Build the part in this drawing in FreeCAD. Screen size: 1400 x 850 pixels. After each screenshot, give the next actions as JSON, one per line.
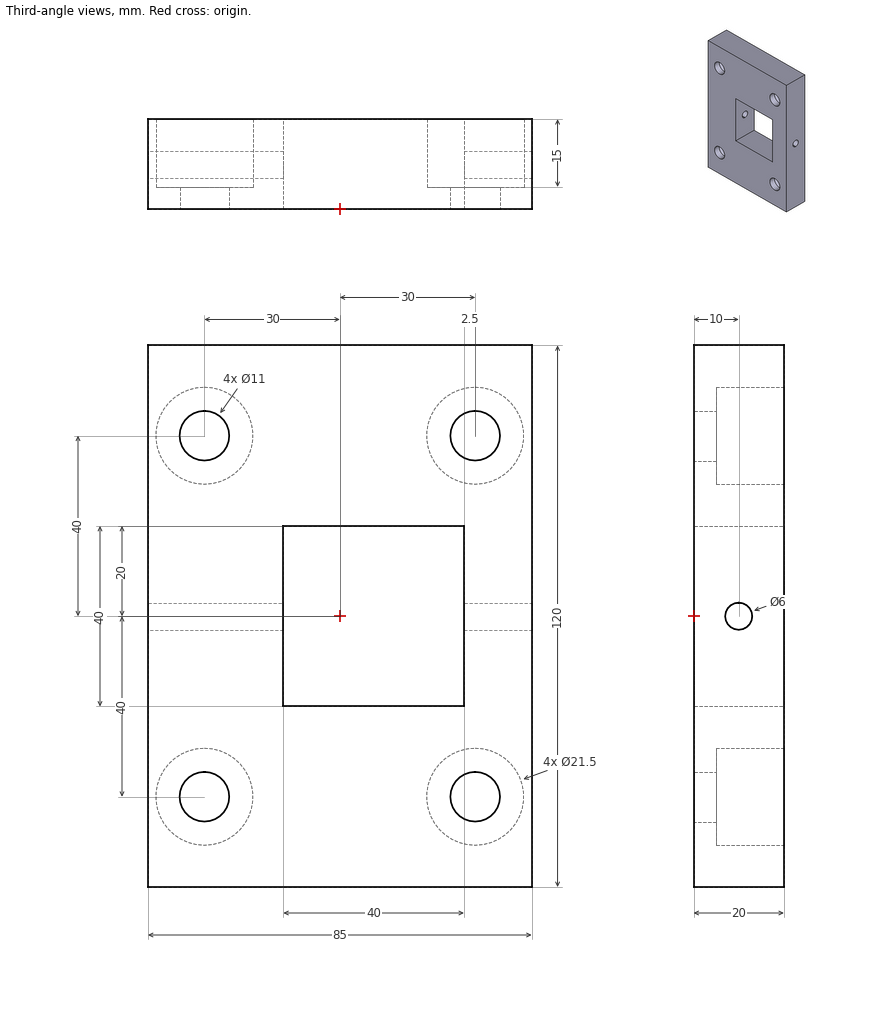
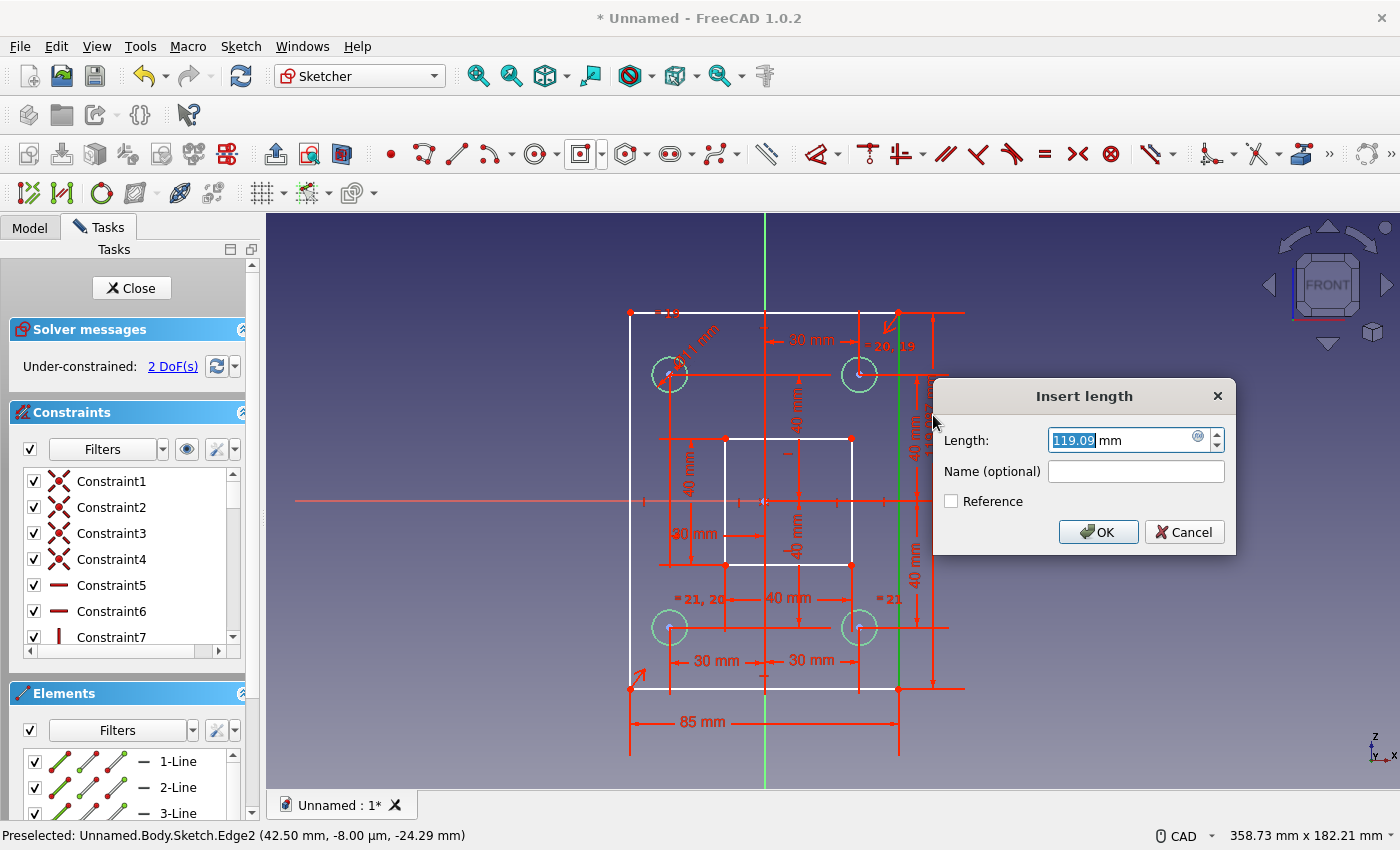
{"action": "type", "text": "120"}
{"action": "key", "text": "Return"}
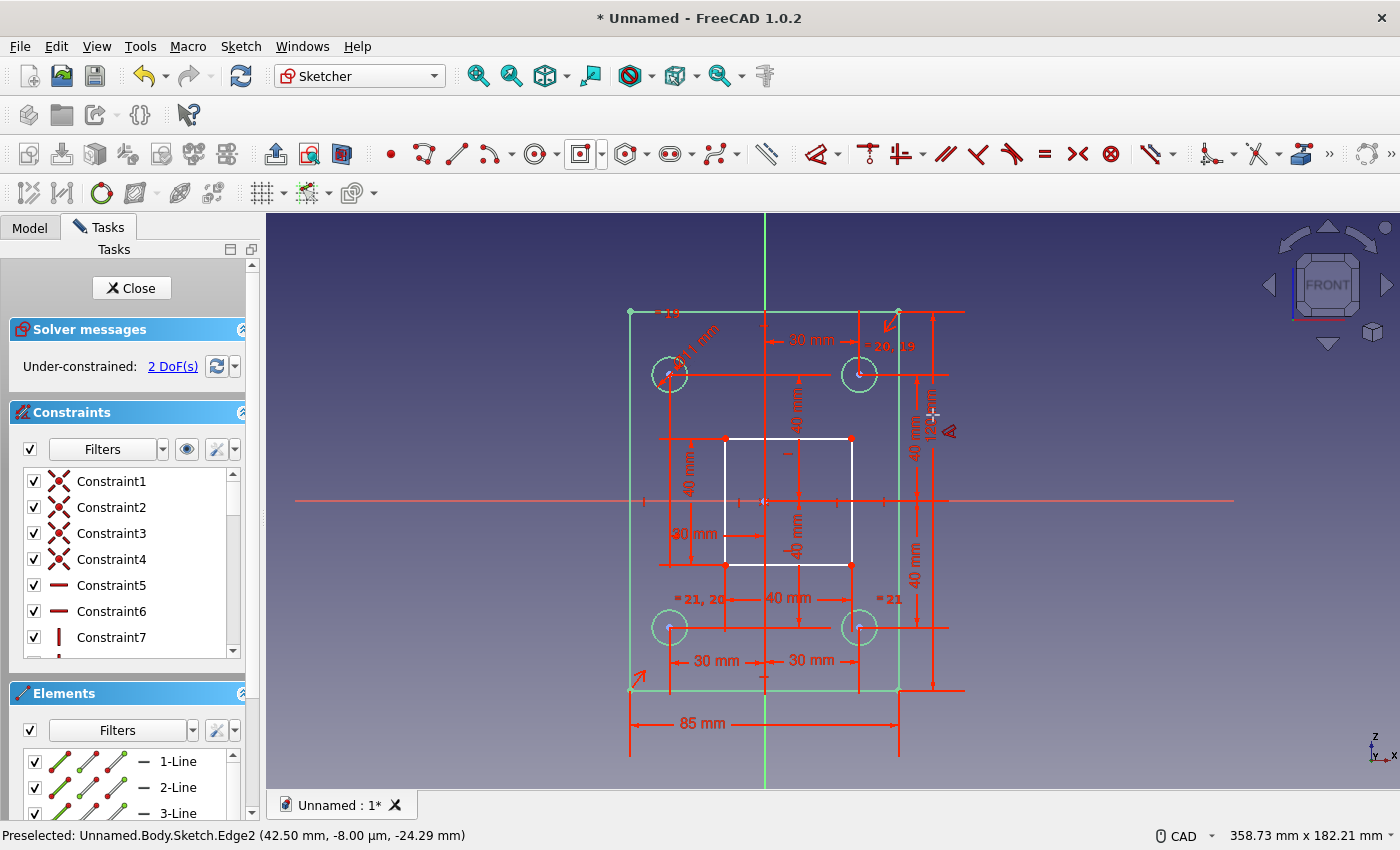
{"action": "left_click", "coordinate": [725, 439]}
{"action": "left_click", "coordinate": [691, 448]}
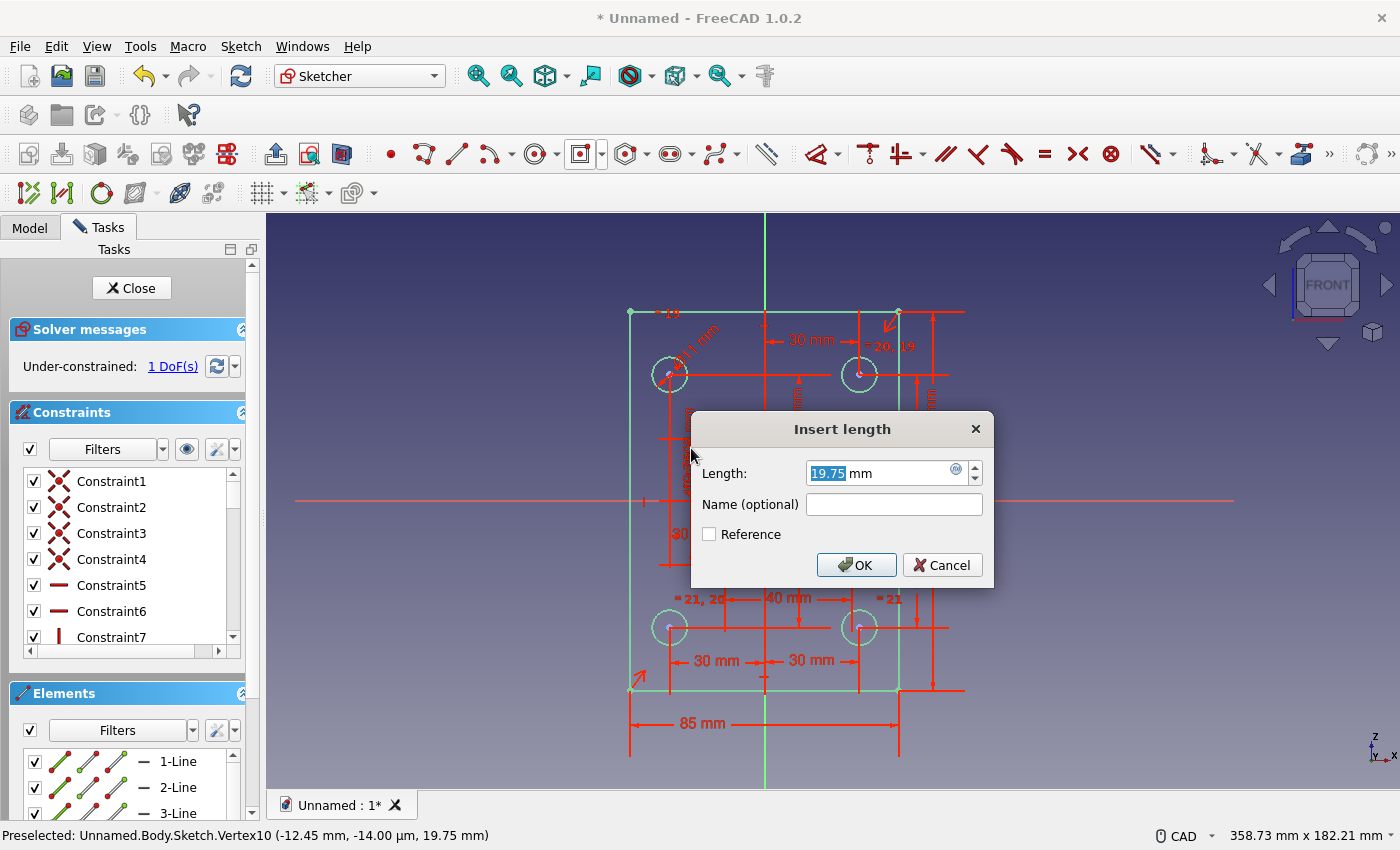
{"action": "type", "text": "20"}
{"action": "key", "text": "Return"}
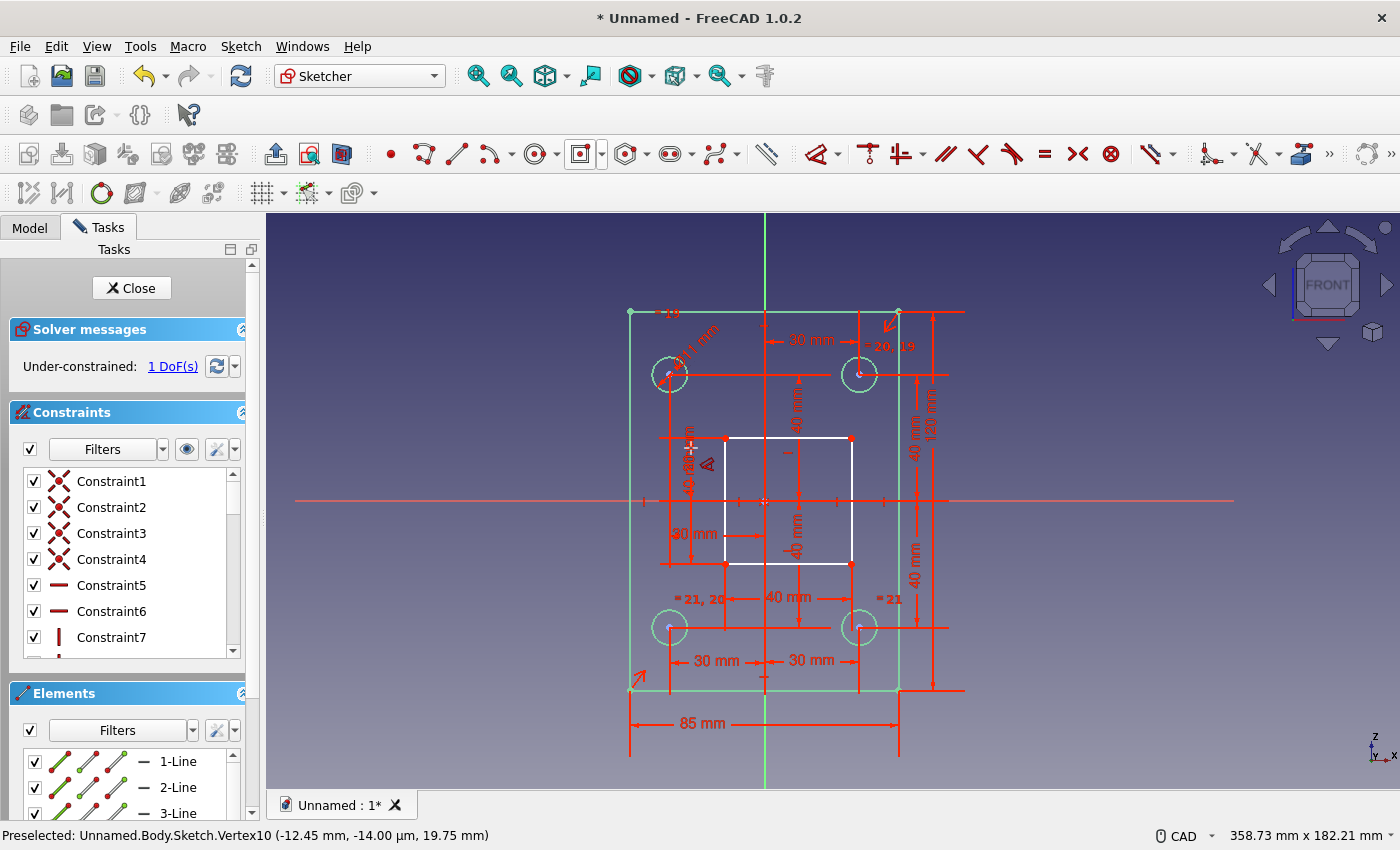
{"action": "scroll", "coordinate": [852, 438], "scroll_direction": "up", "scroll_amount": 9}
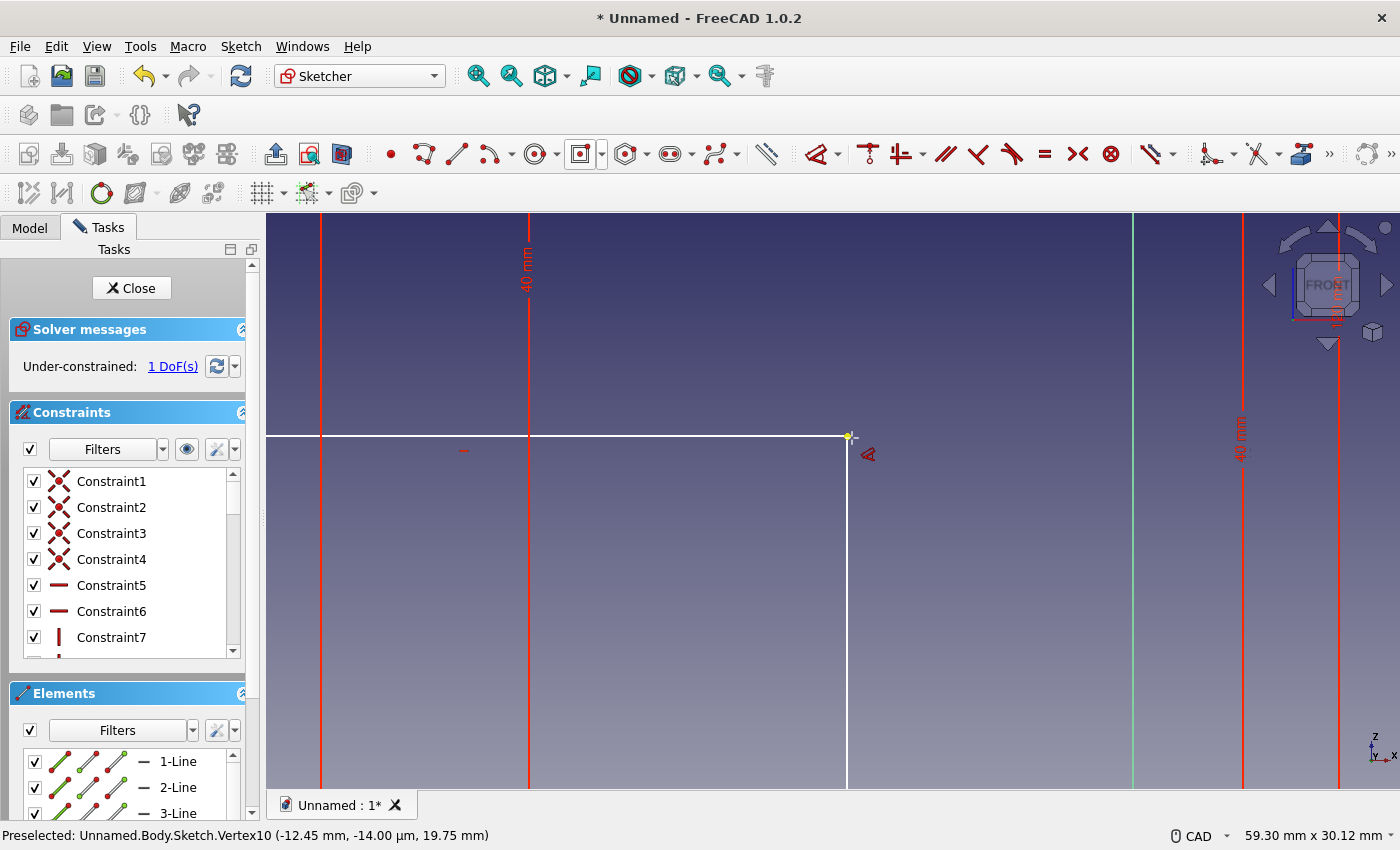
{"action": "left_click", "coordinate": [847, 436]}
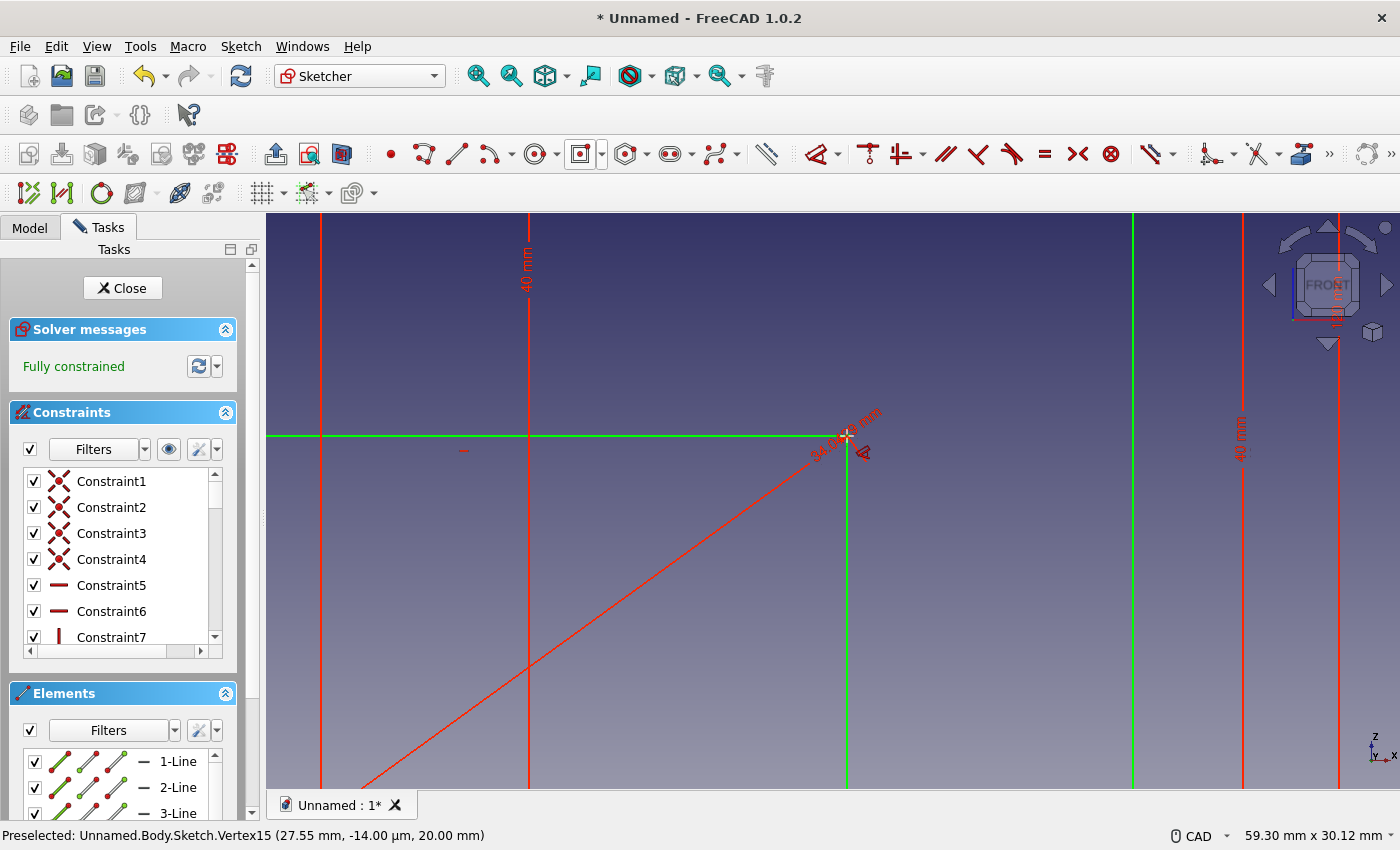
{"action": "scroll", "coordinate": [852, 438], "scroll_direction": "down", "scroll_amount": 9}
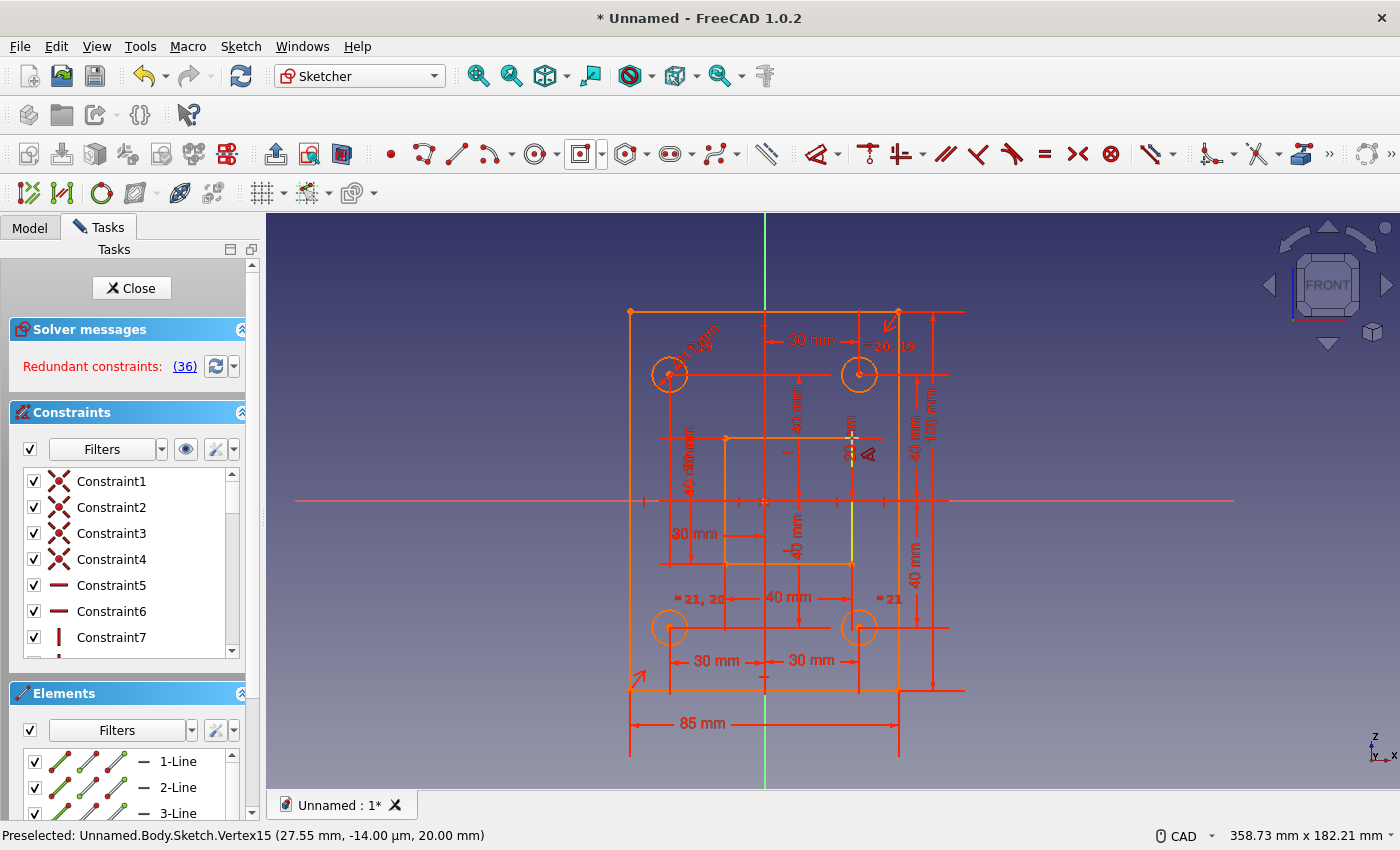
{"action": "scroll", "coordinate": [859, 375], "scroll_direction": "up", "scroll_amount": 9}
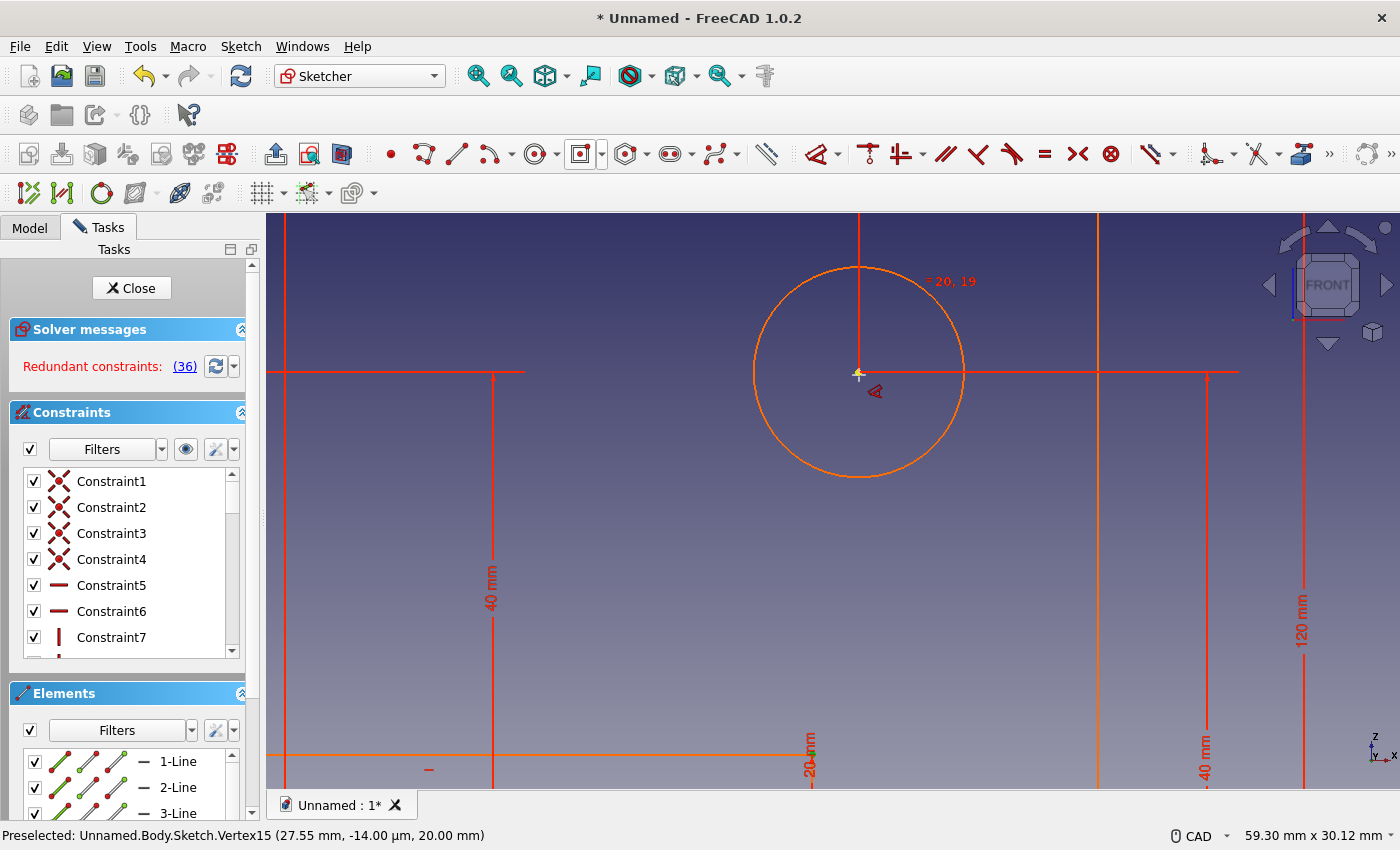
{"action": "left_click", "coordinate": [859, 372]}
{"action": "left_click", "coordinate": [835, 338]}